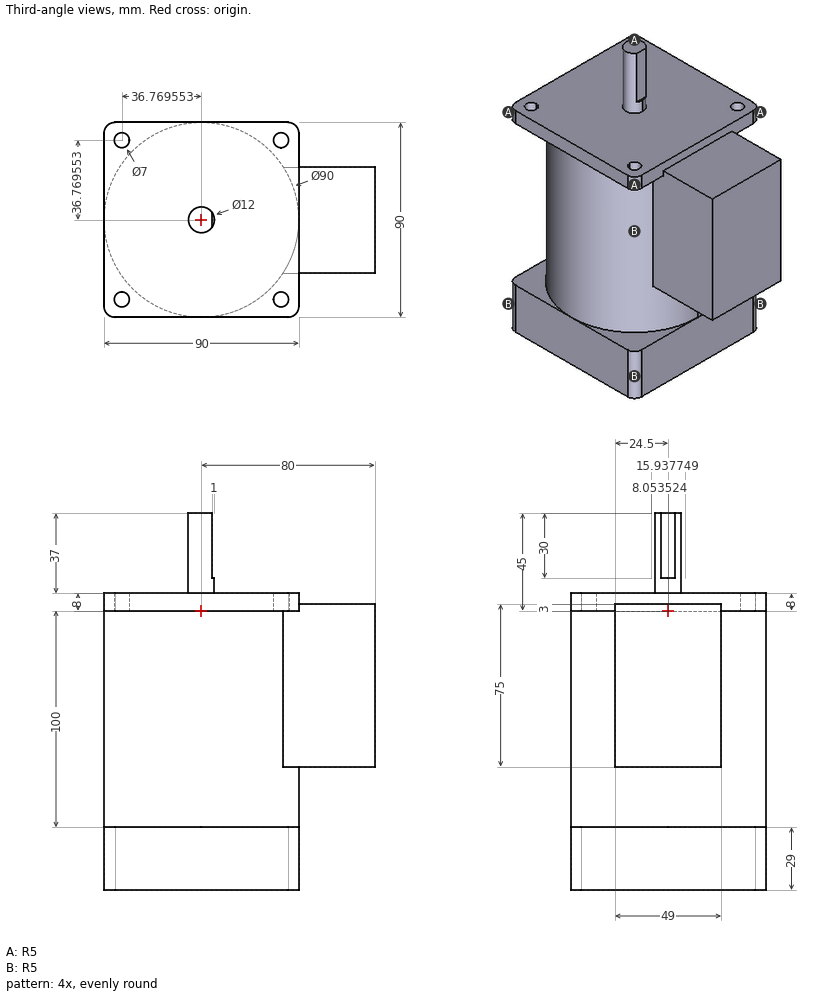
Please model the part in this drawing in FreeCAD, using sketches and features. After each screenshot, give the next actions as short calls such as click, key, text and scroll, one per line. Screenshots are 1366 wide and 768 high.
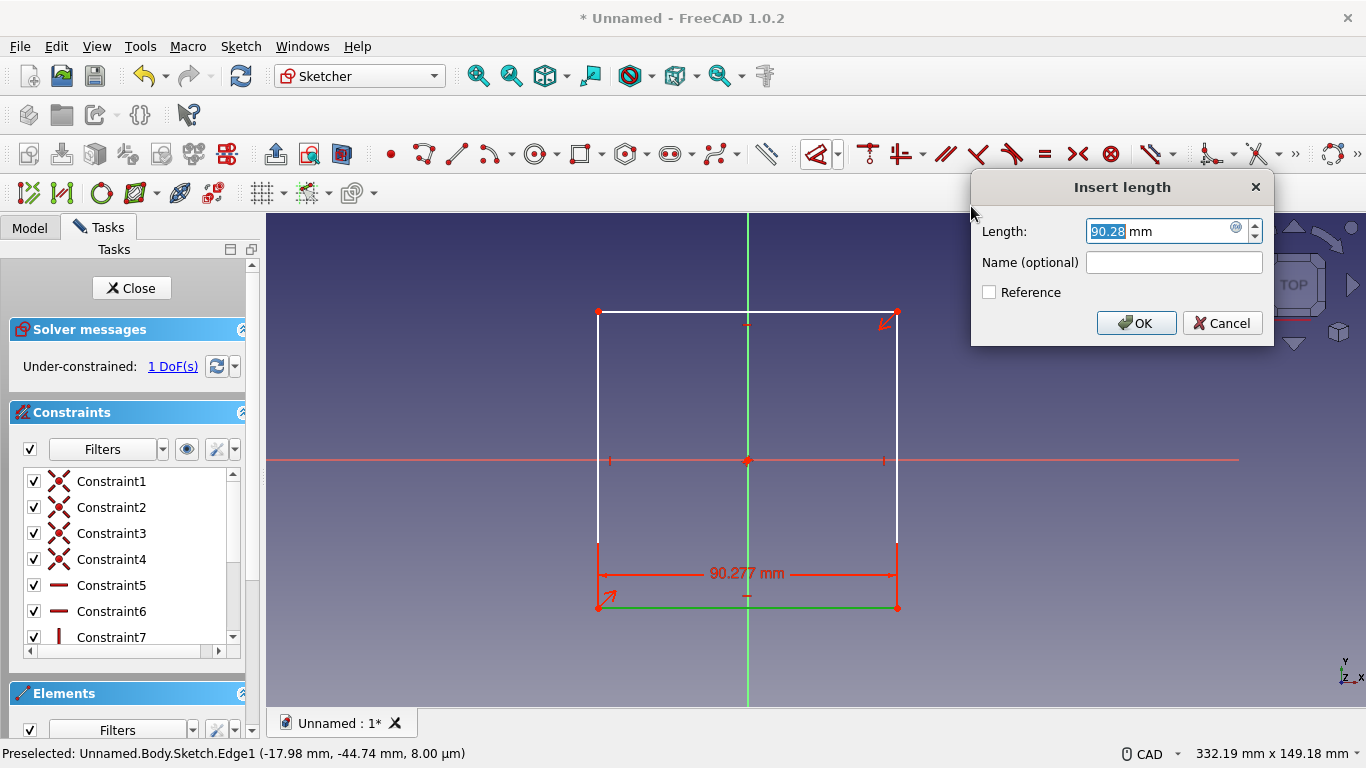
text(90)
key(Return)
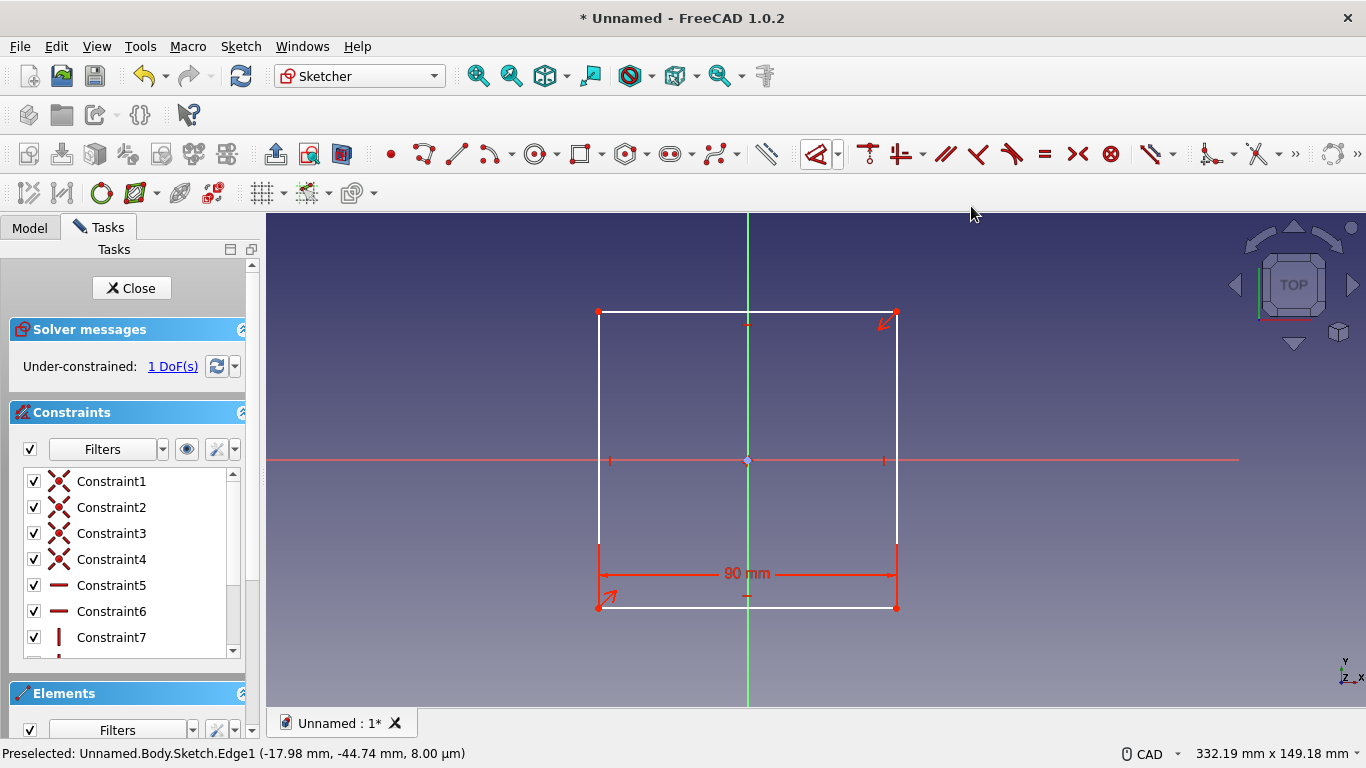
click(897, 519)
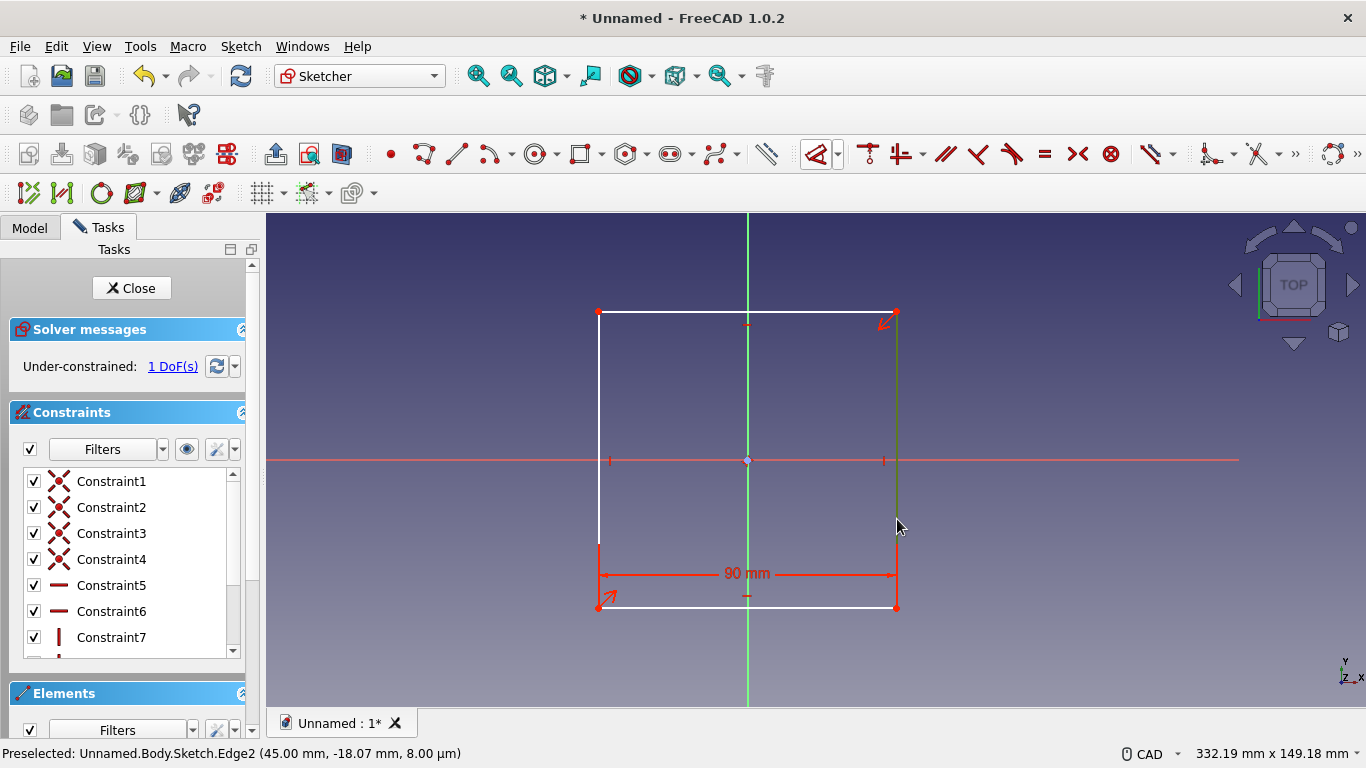
click(838, 154)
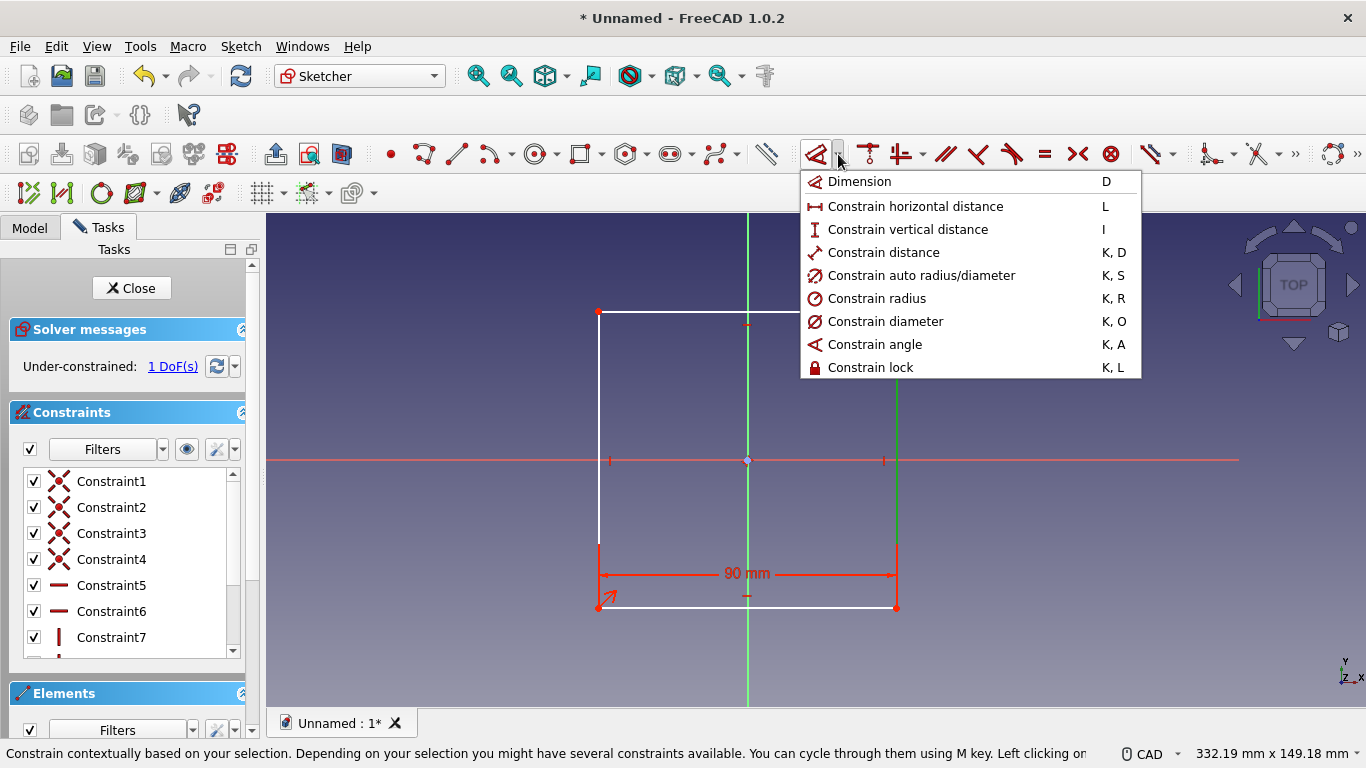
click(971, 230)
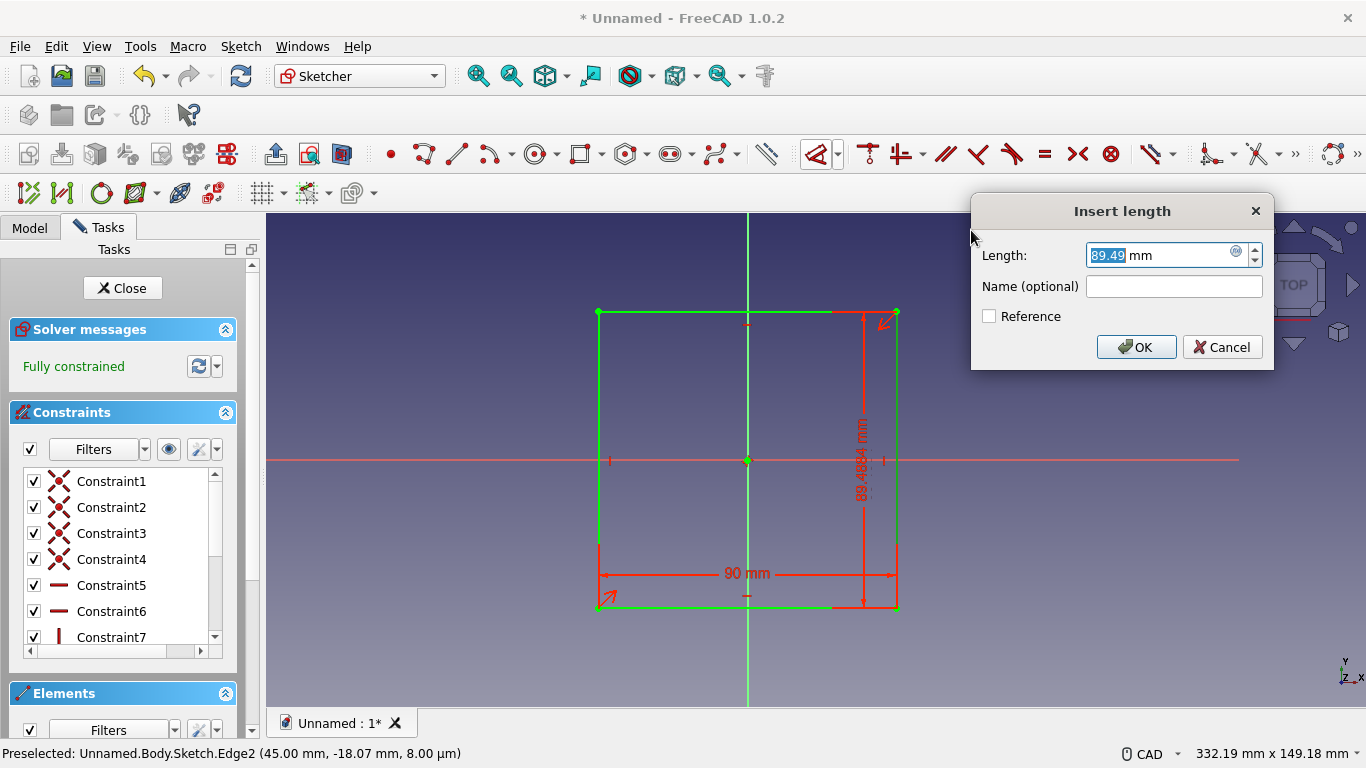
text(90)
key(Return)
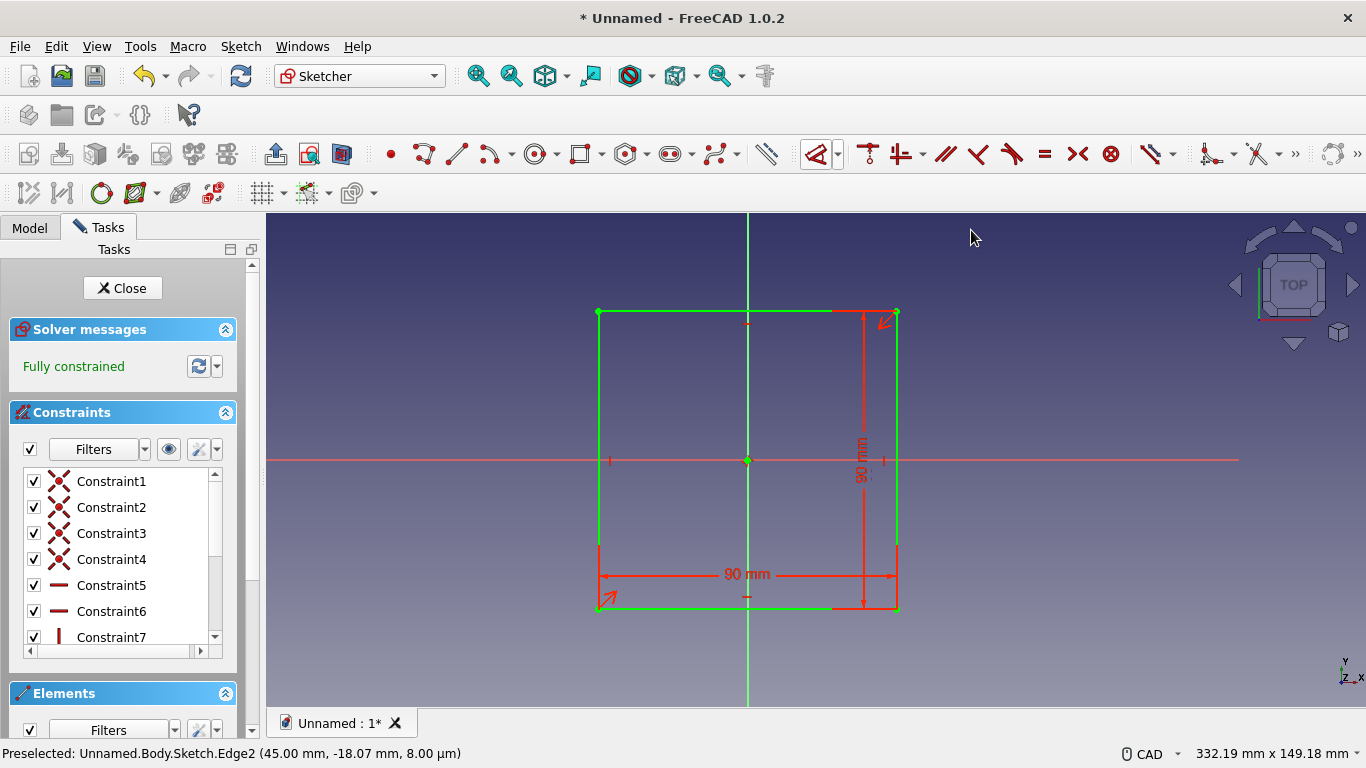
click(123, 288)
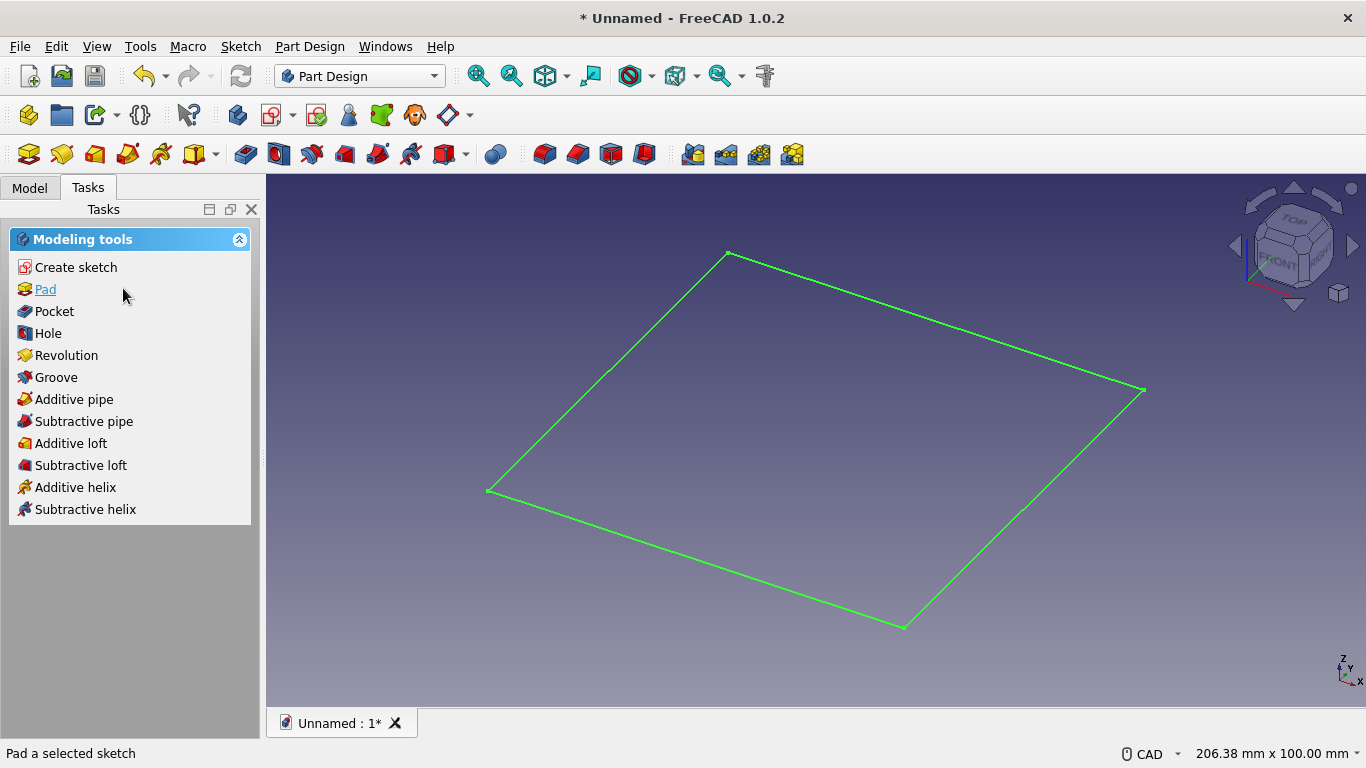
click(29, 154)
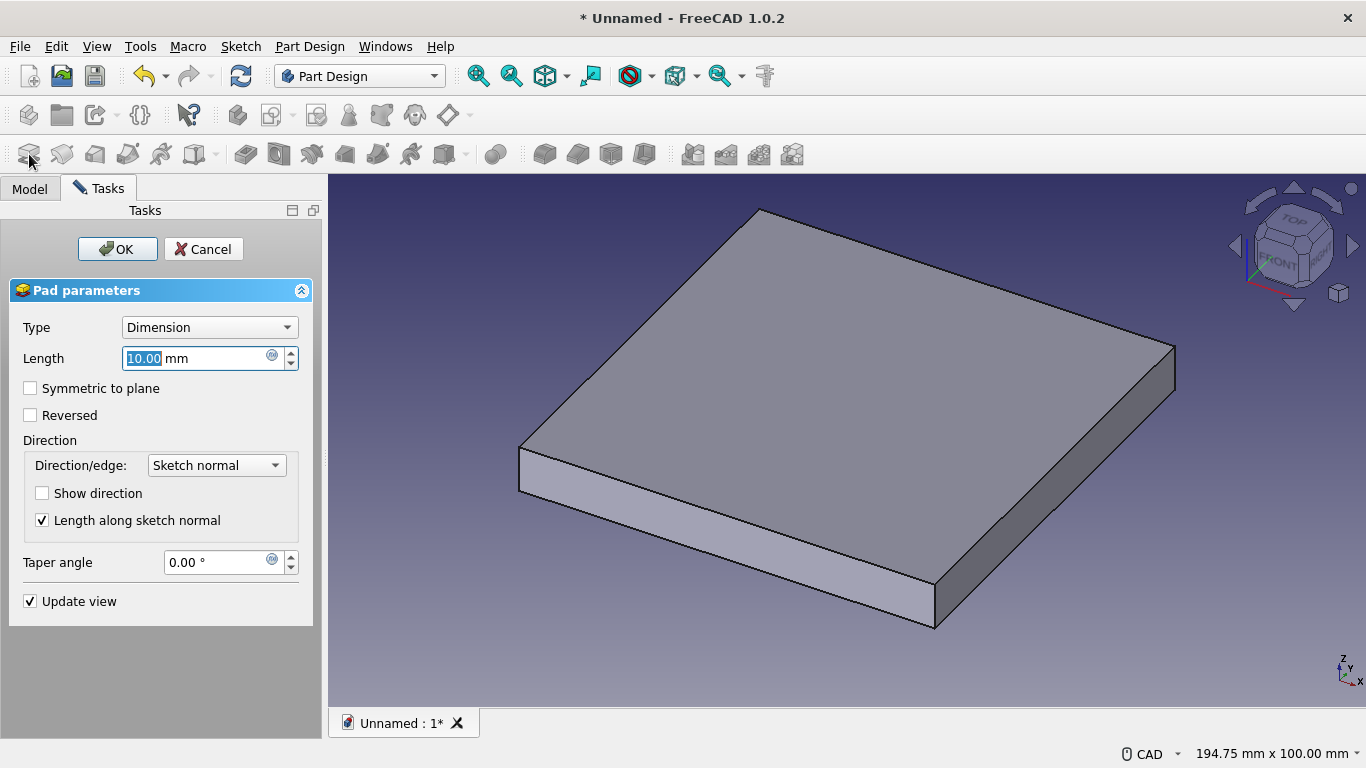
text(8)
key(Tab)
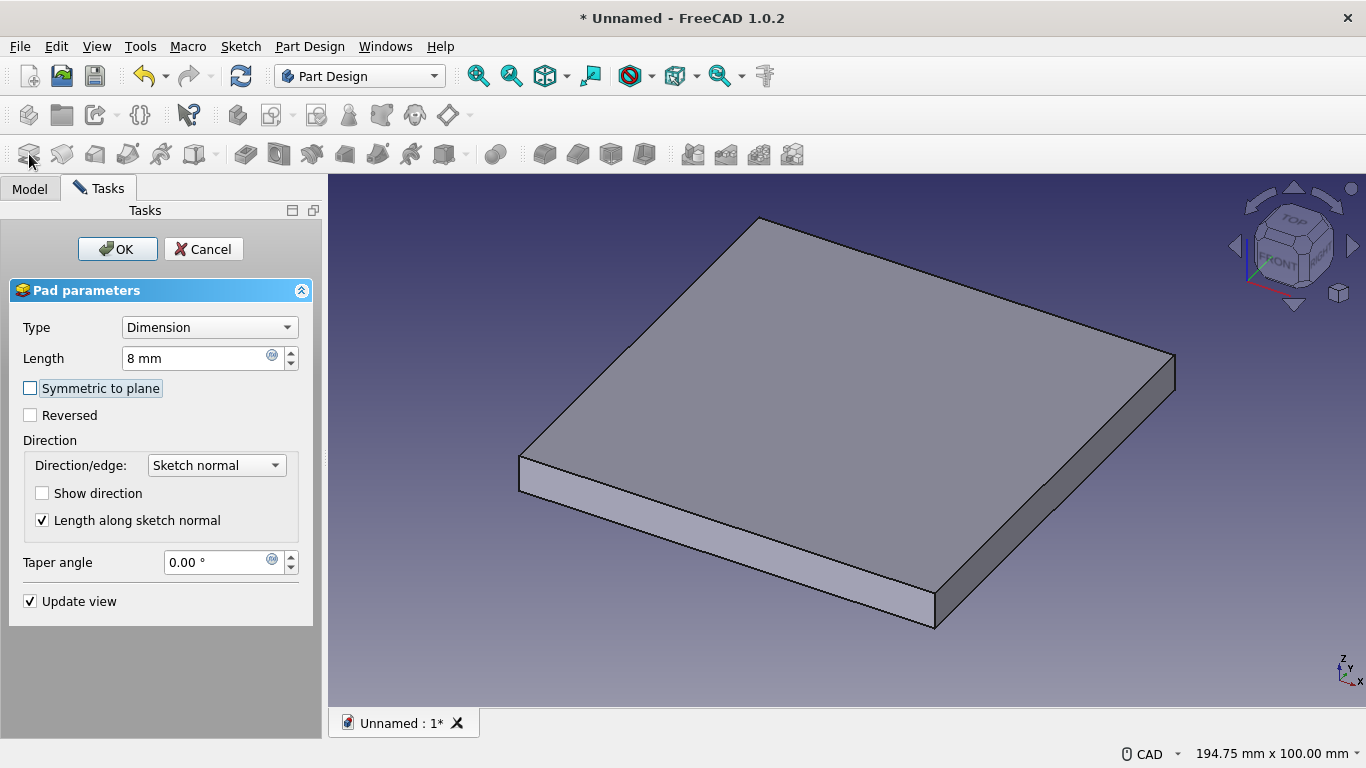
click(118, 249)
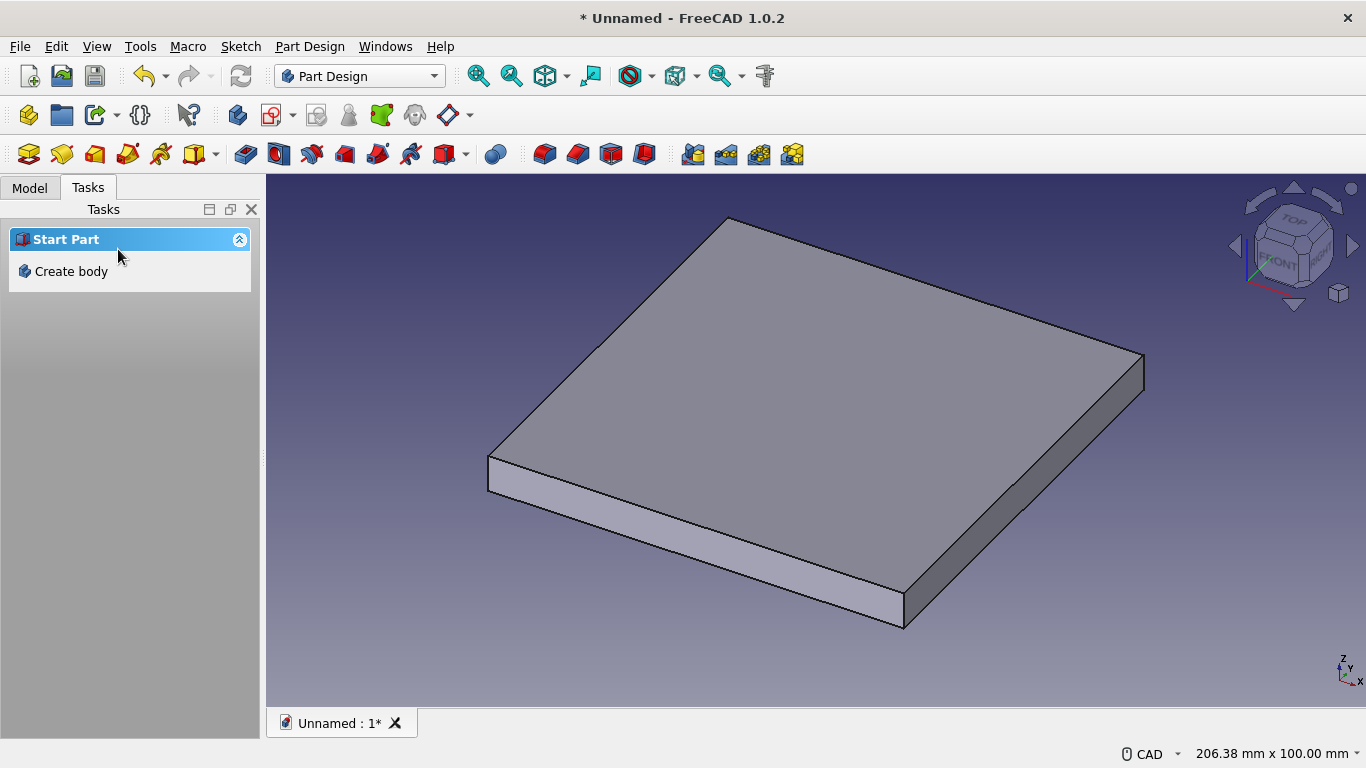
click(270, 116)